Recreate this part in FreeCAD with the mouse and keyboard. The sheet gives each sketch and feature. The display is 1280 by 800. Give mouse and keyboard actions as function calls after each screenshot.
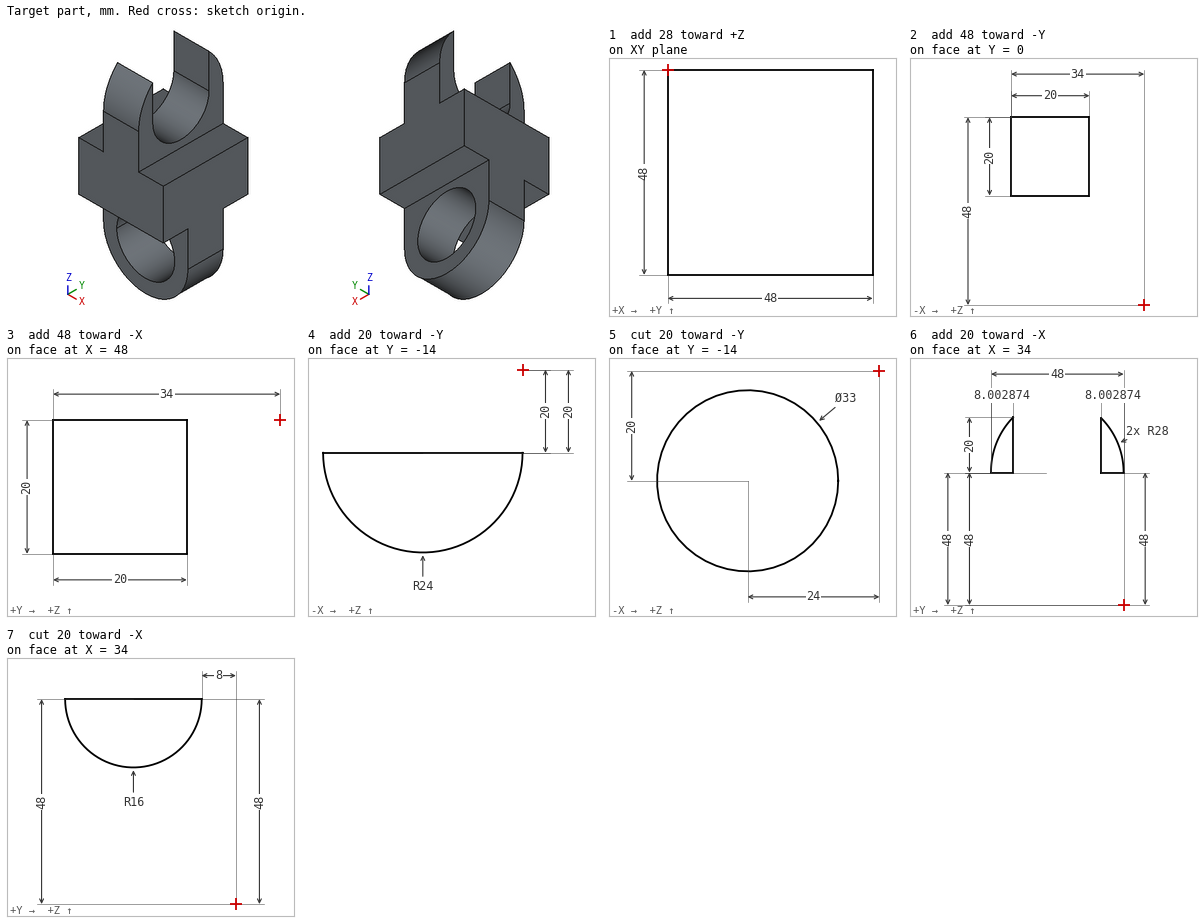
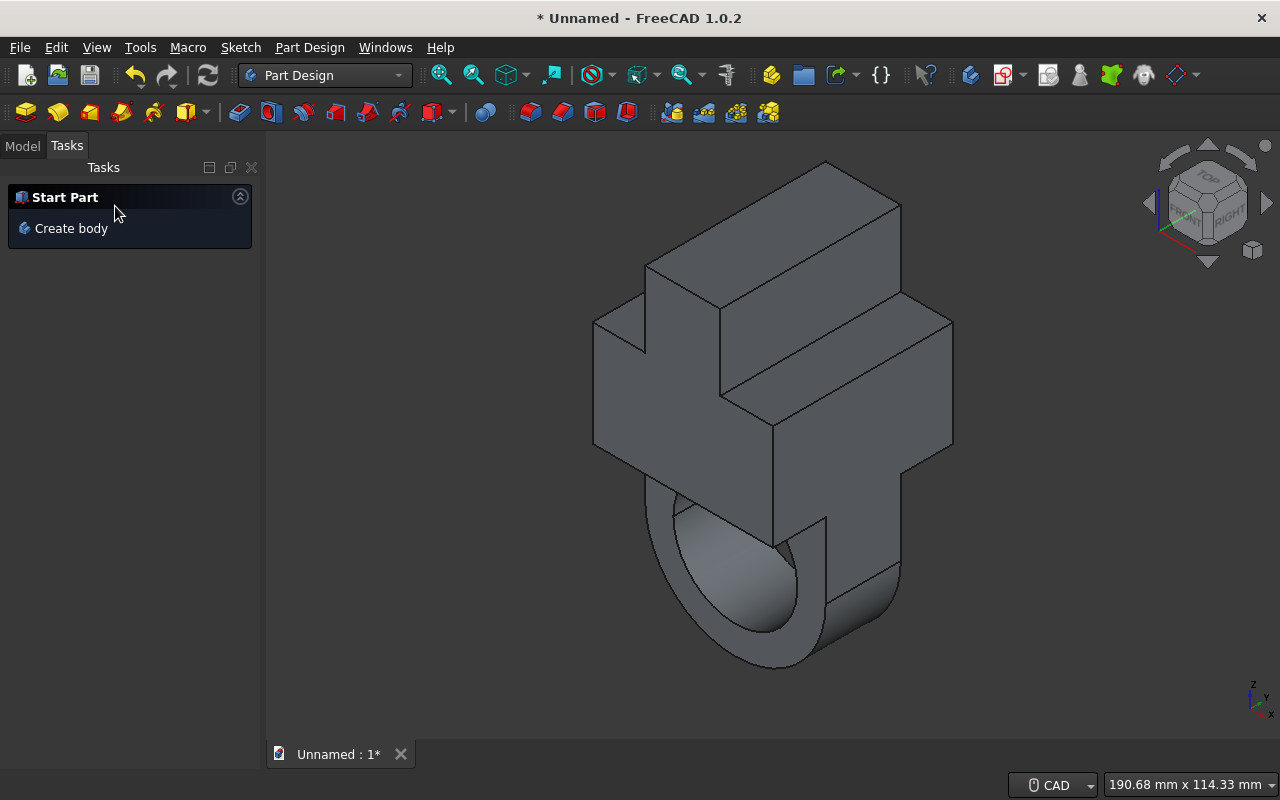
click(442, 76)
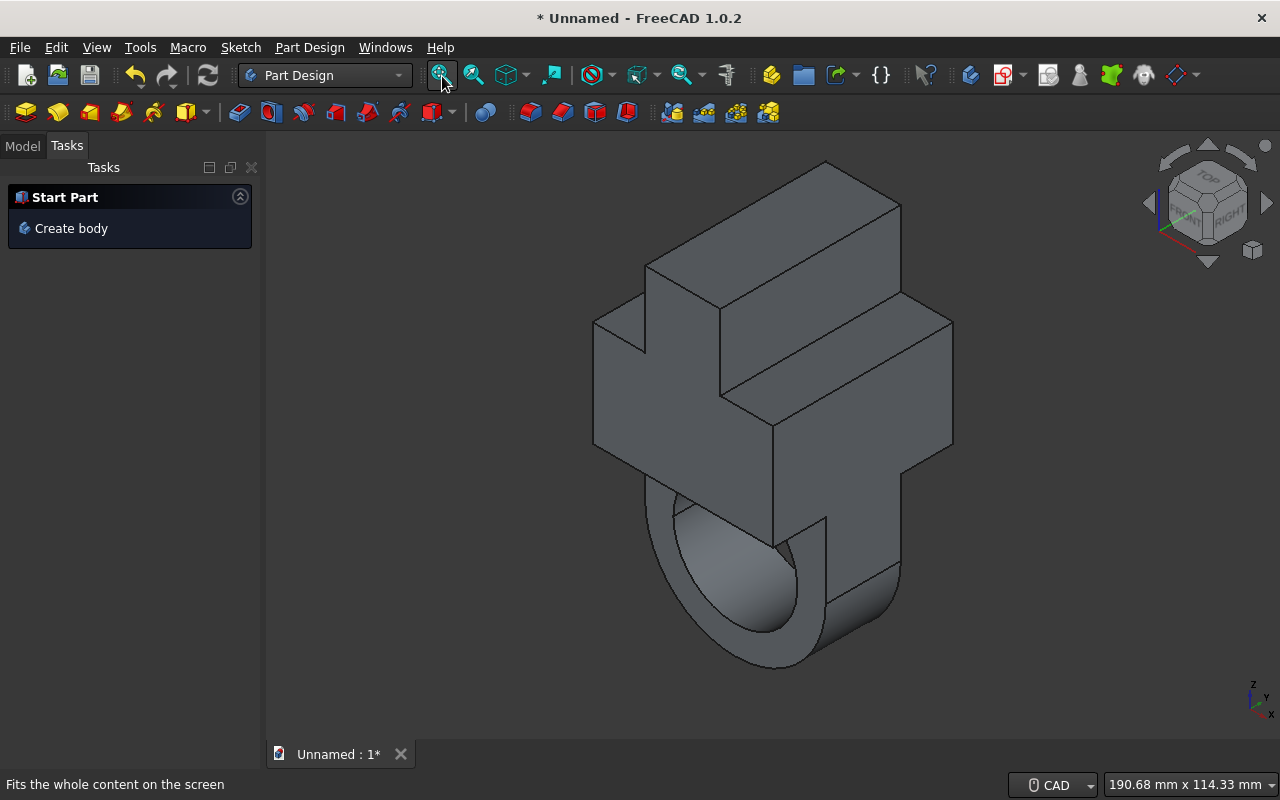
click(836, 285)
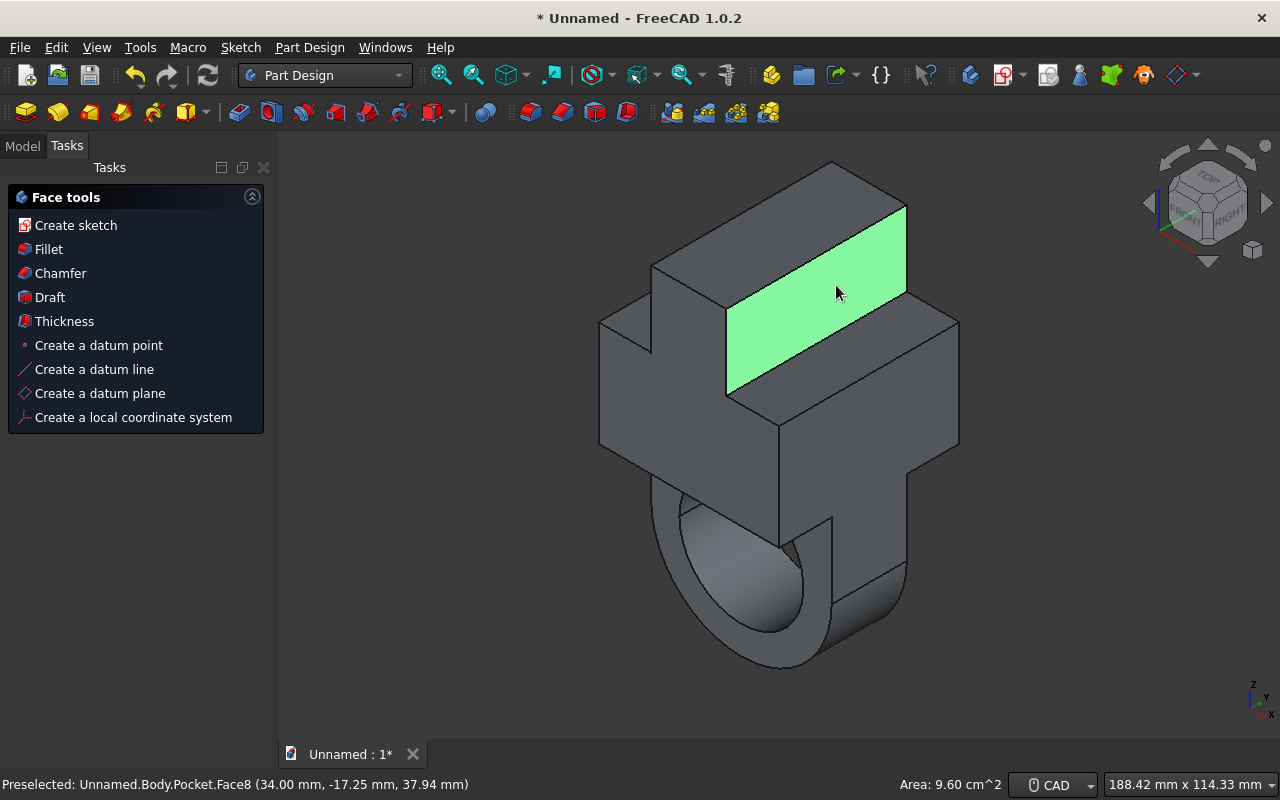
click(1004, 76)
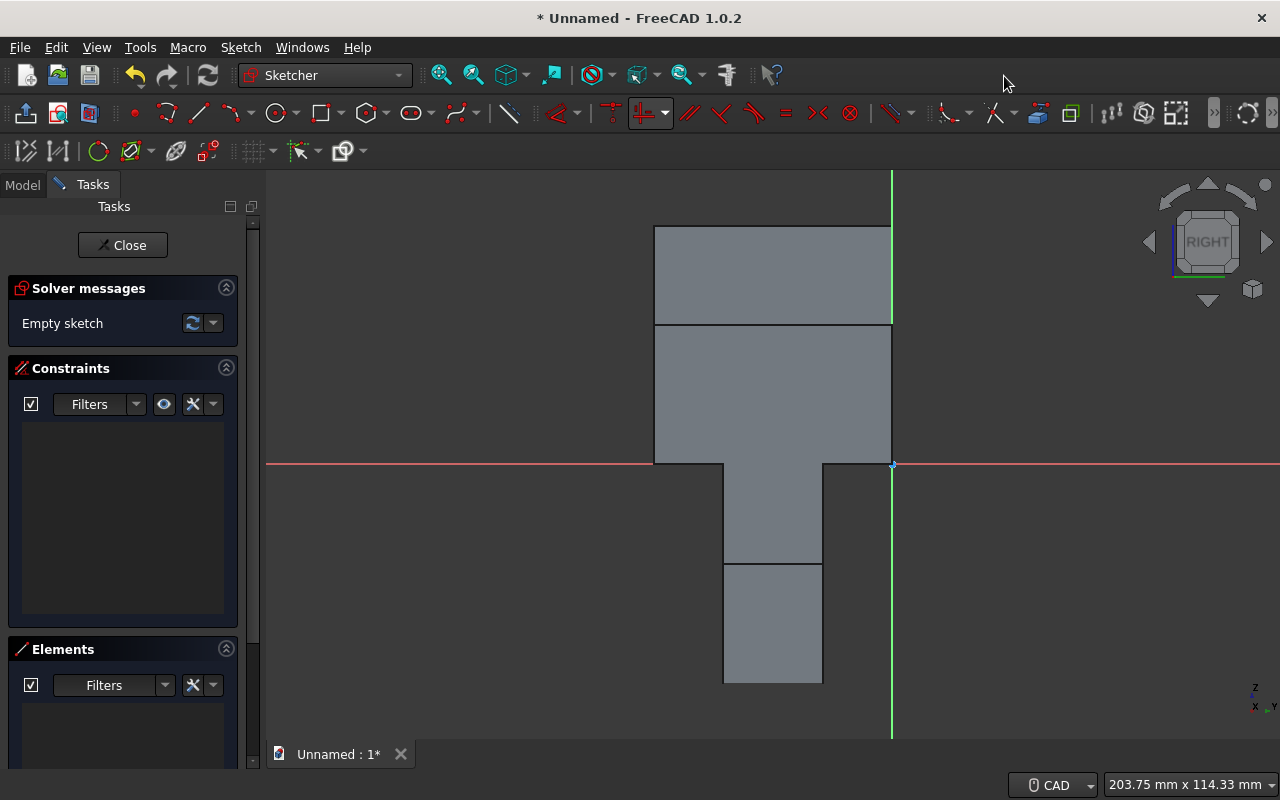
key(q)
key(s)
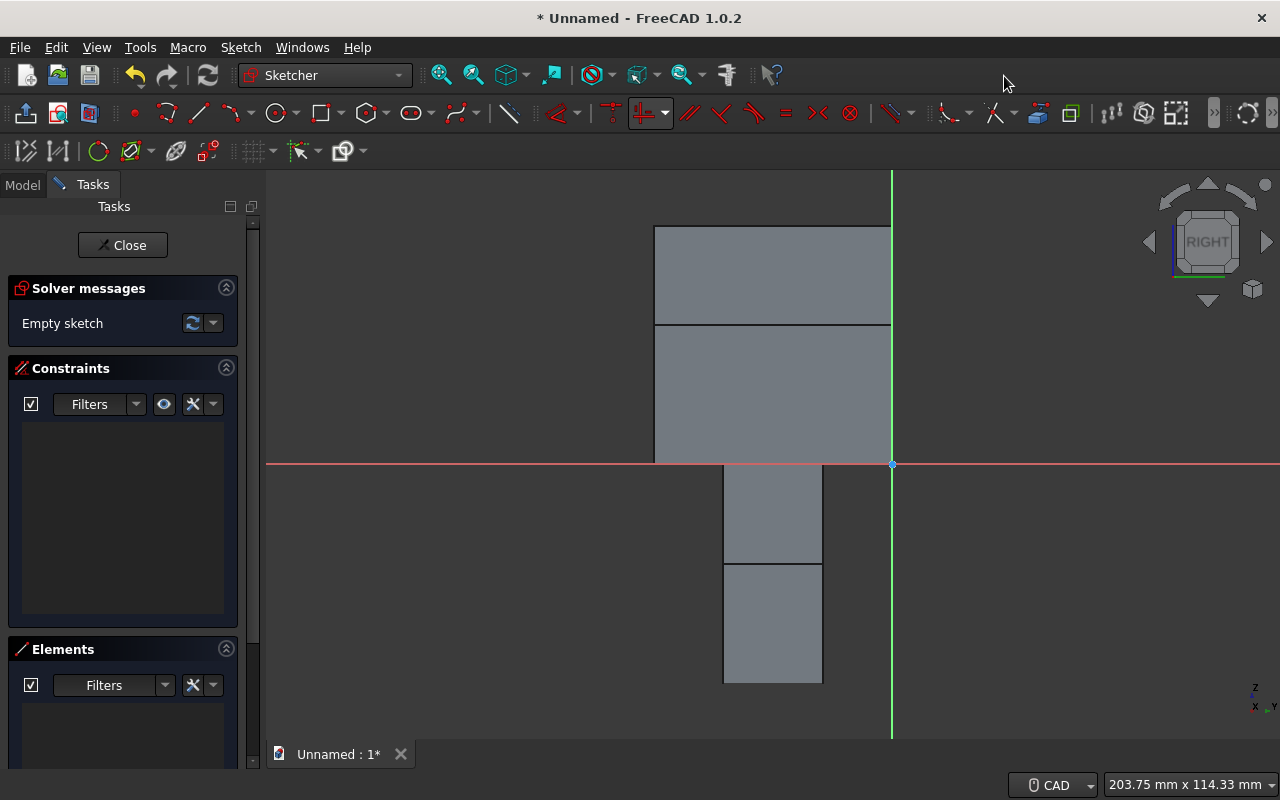
scroll(395, 711, down, 1)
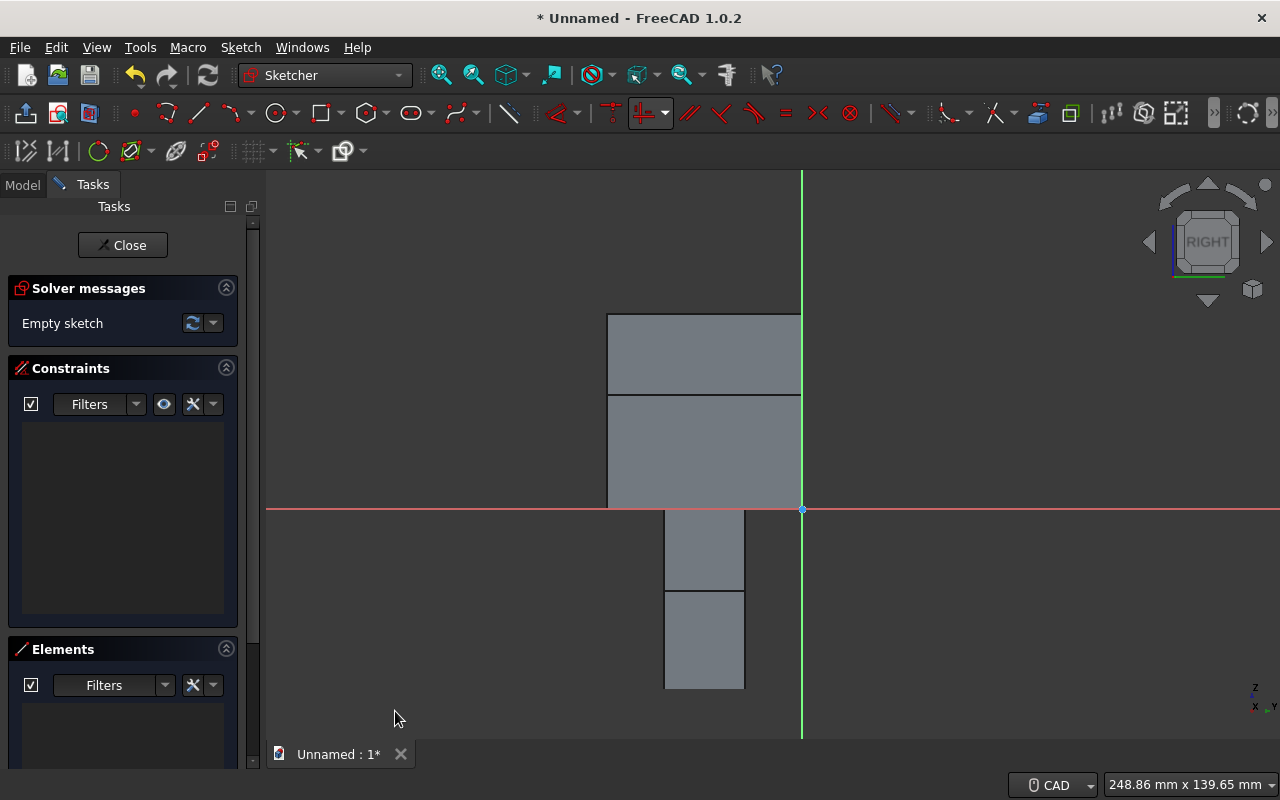
key(g)
key(m)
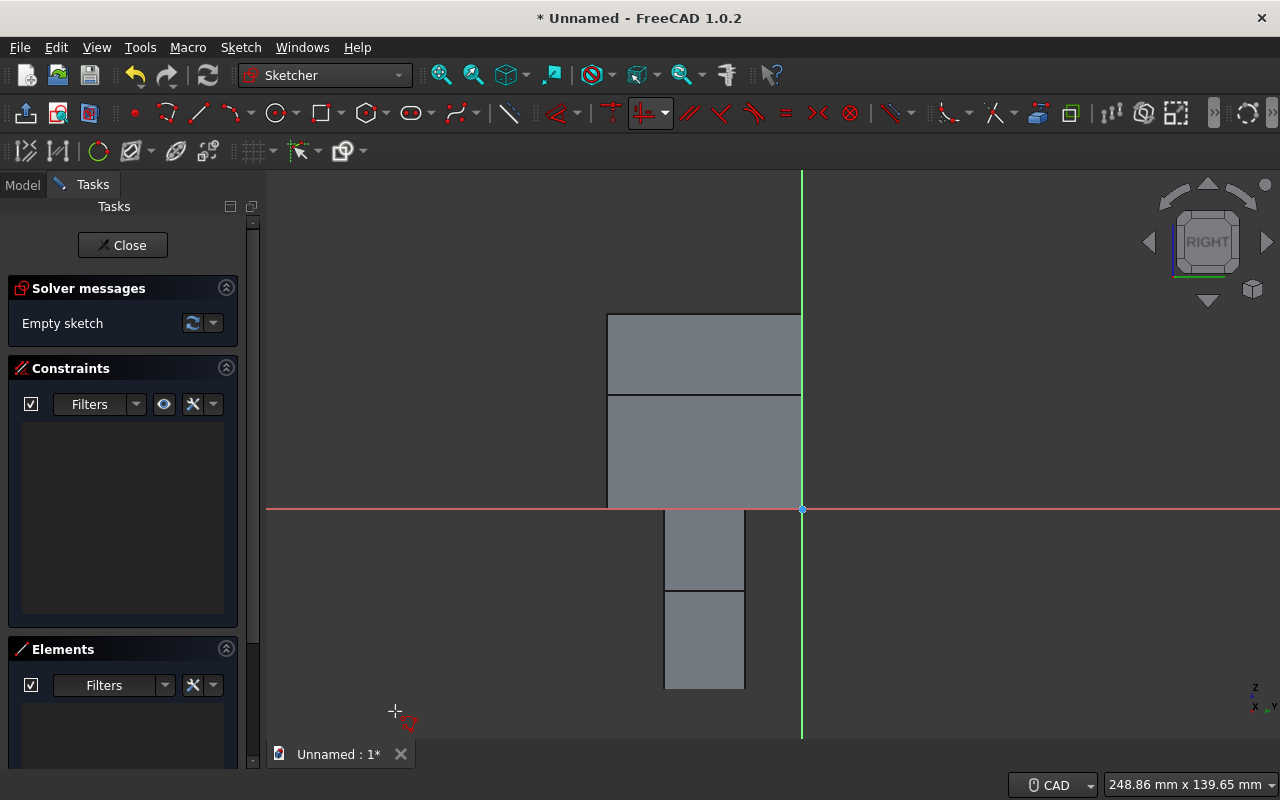
click(770, 234)
click(770, 314)
click(802, 314)
right_click(802, 314)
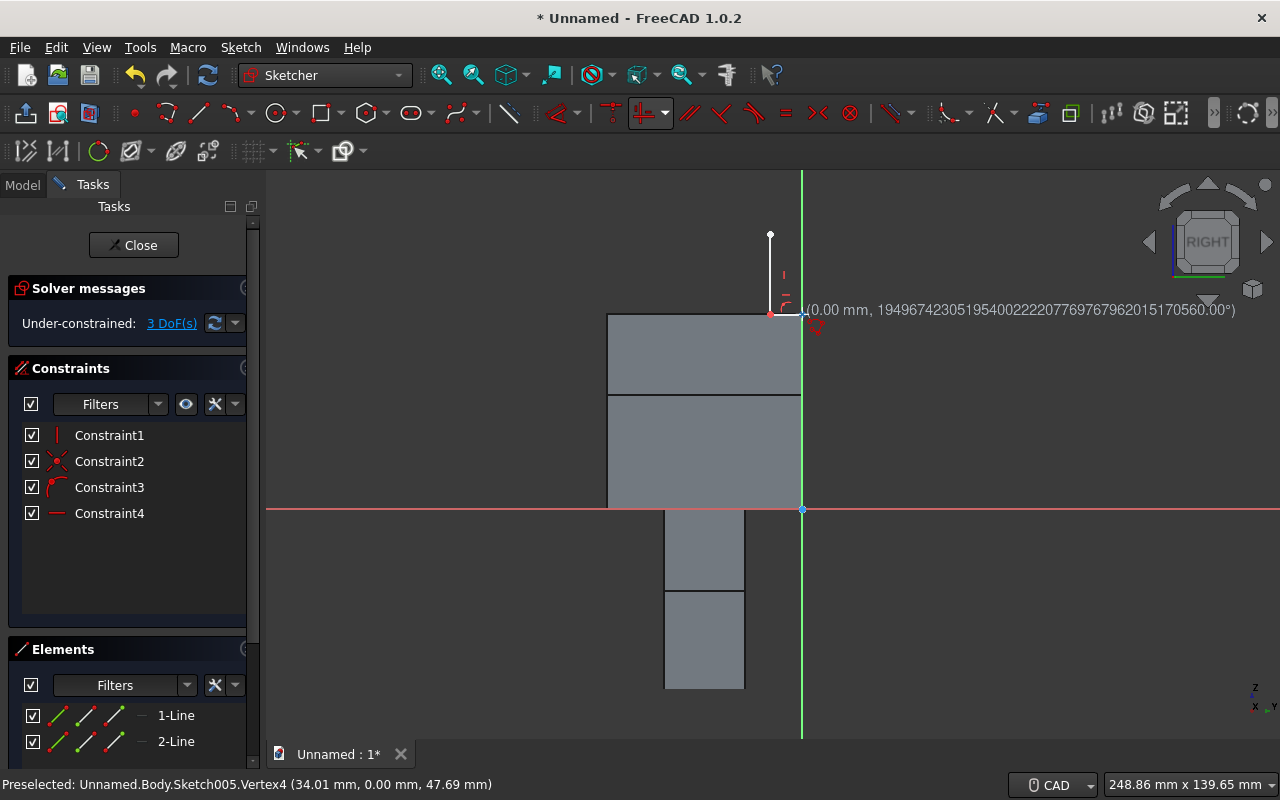
click(232, 114)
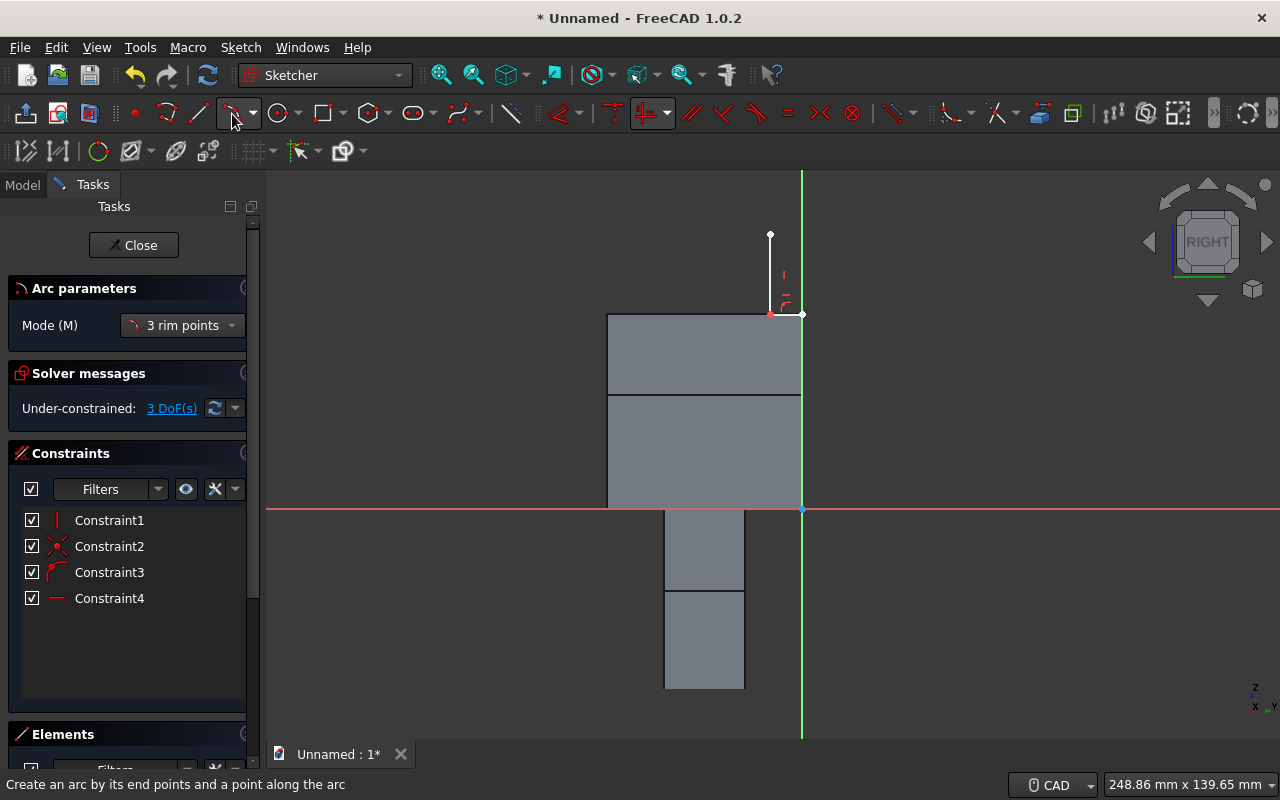
click(802, 315)
click(770, 235)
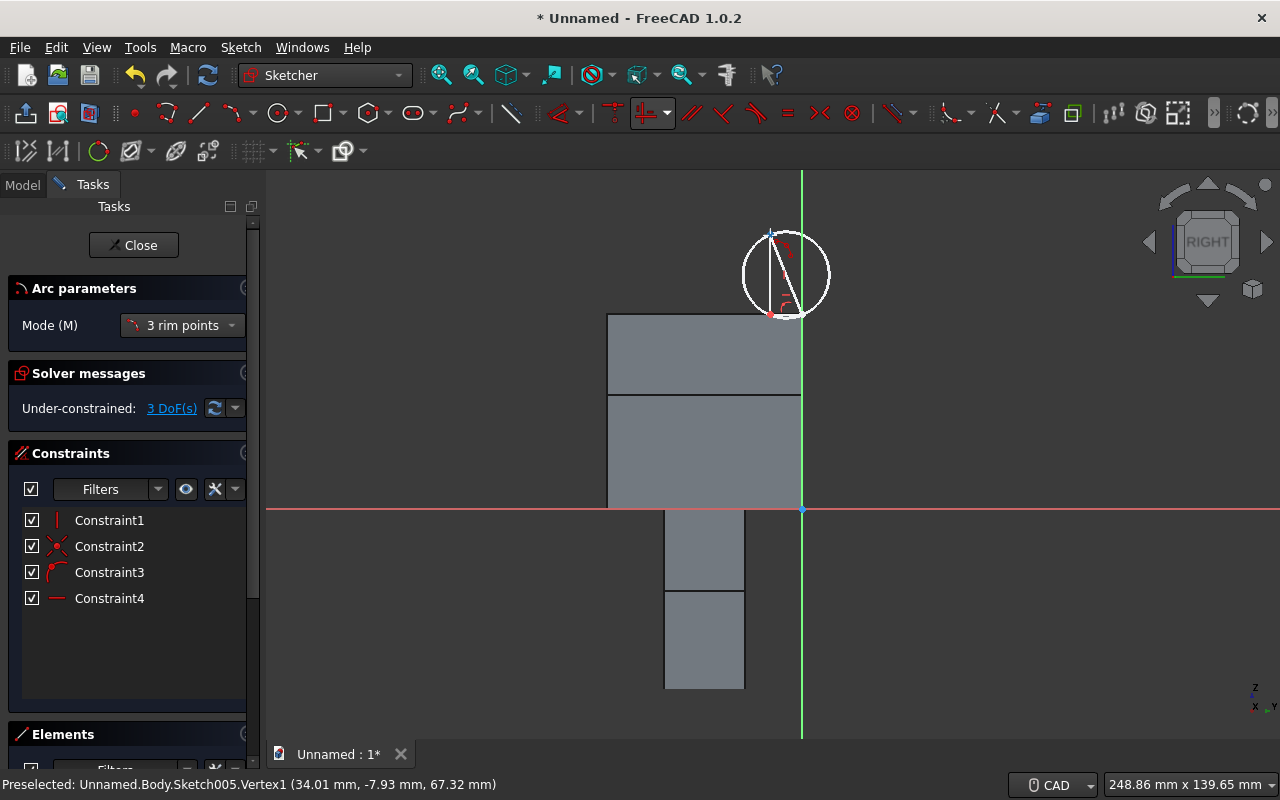
scroll(794, 271, up, 4)